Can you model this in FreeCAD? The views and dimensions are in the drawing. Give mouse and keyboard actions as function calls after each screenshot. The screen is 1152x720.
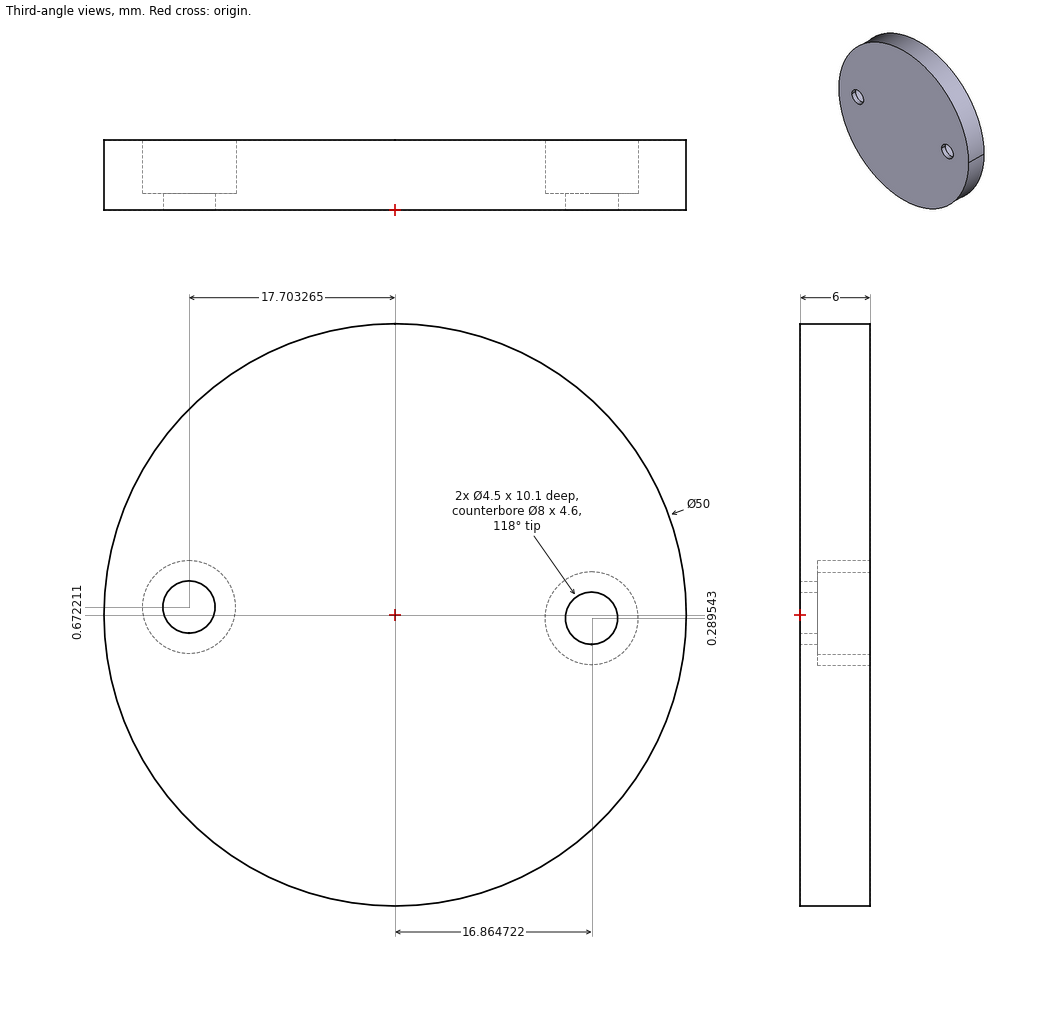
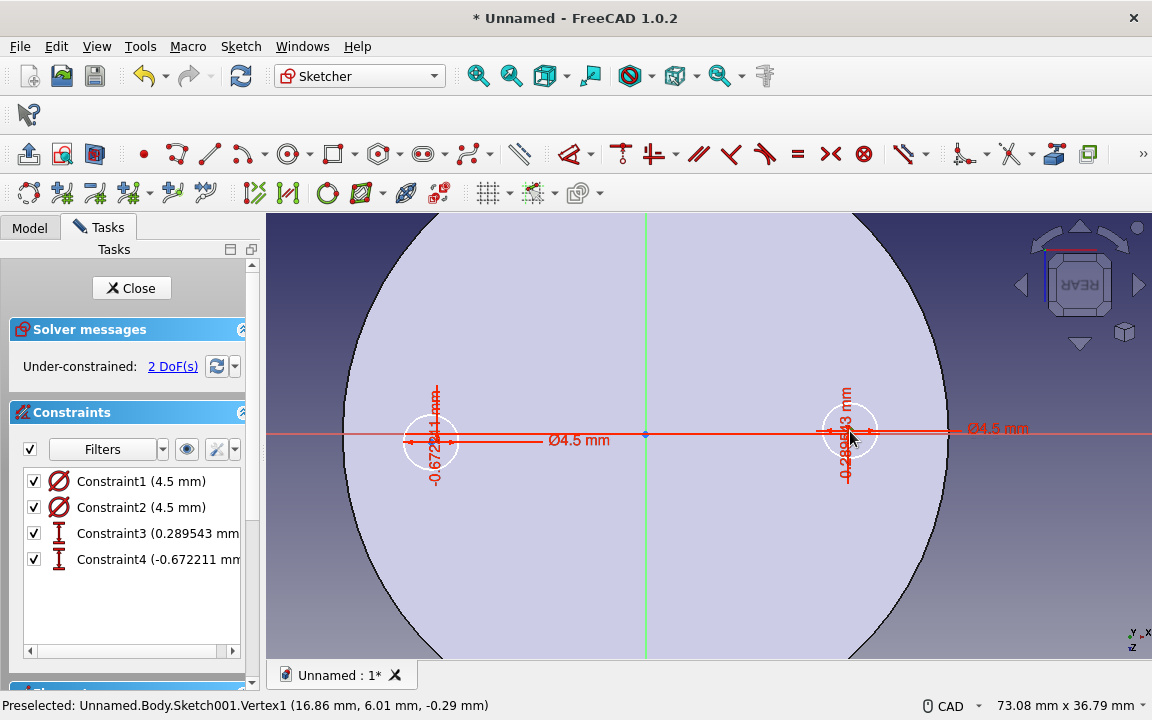
click(590, 154)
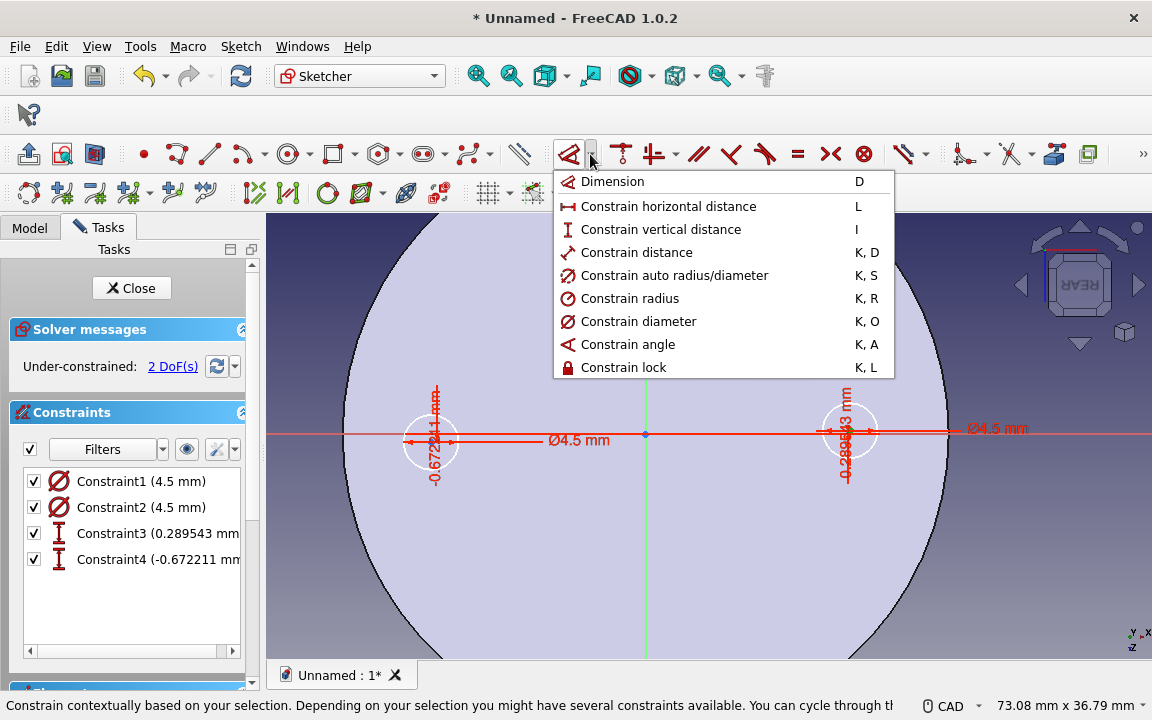
click(724, 206)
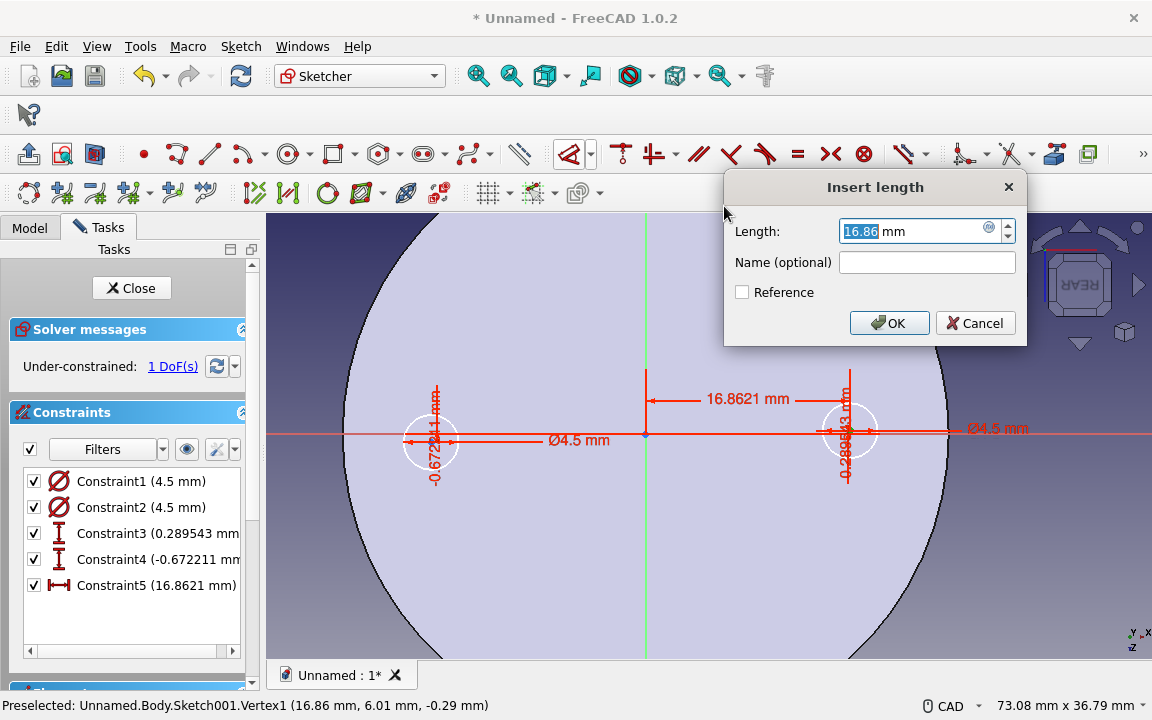
text(16.864722)
key(Return)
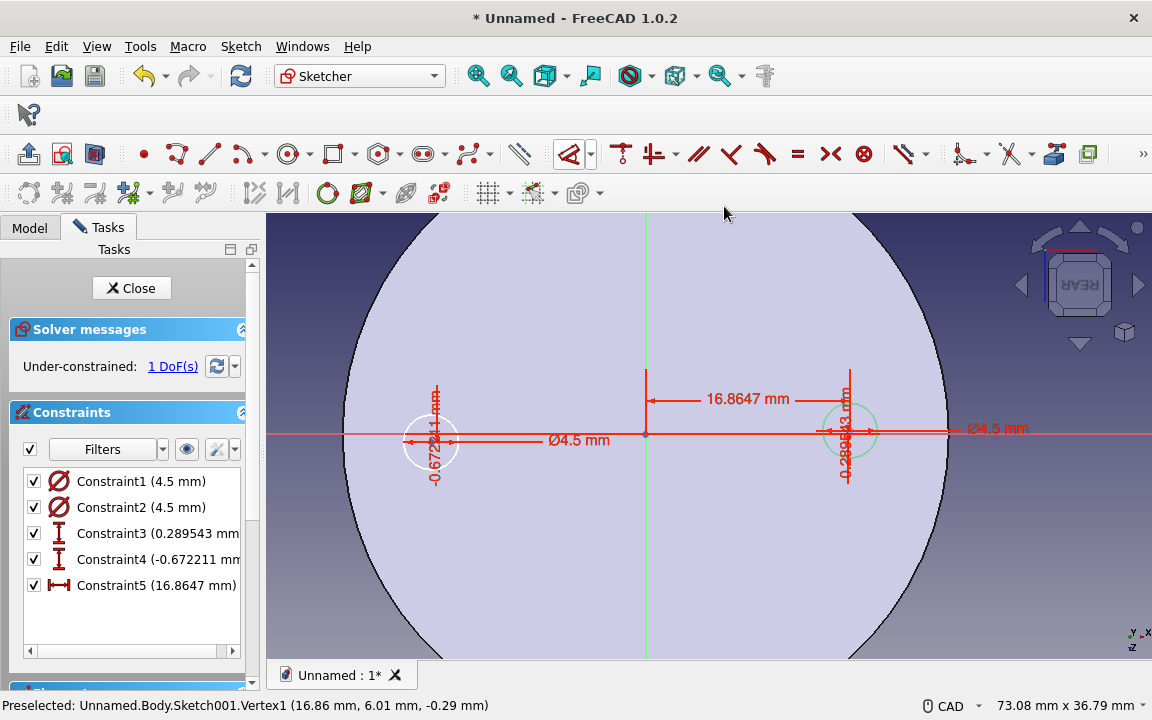
click(431, 442)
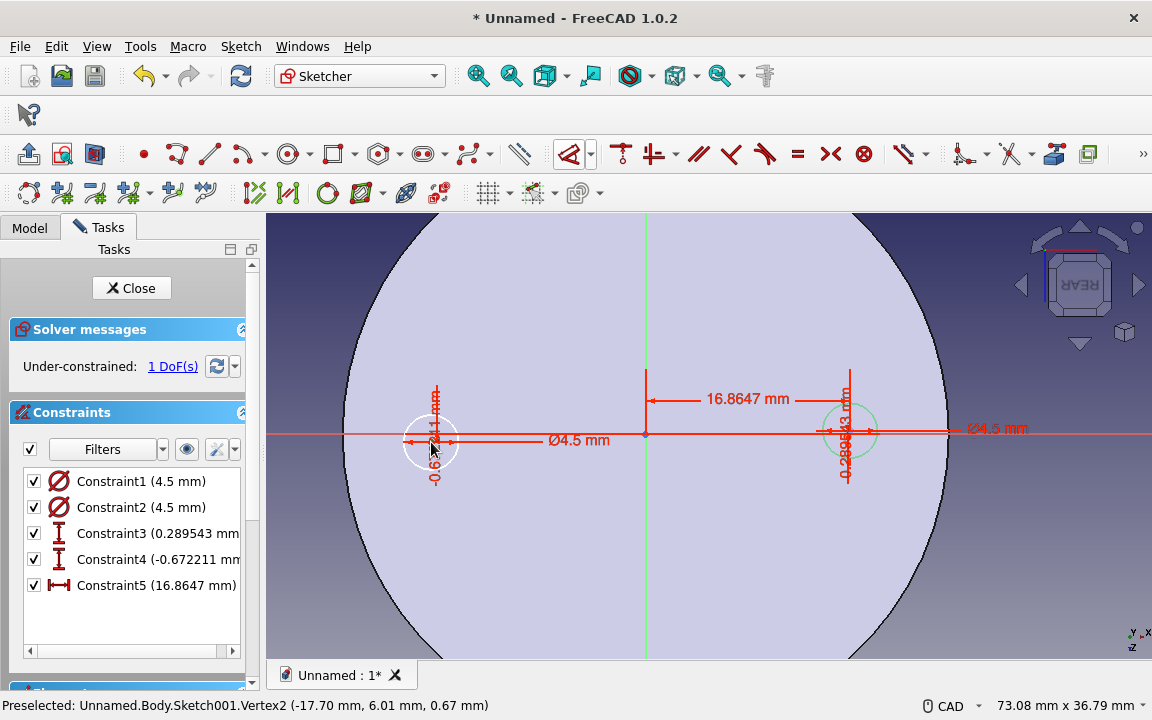
click(590, 154)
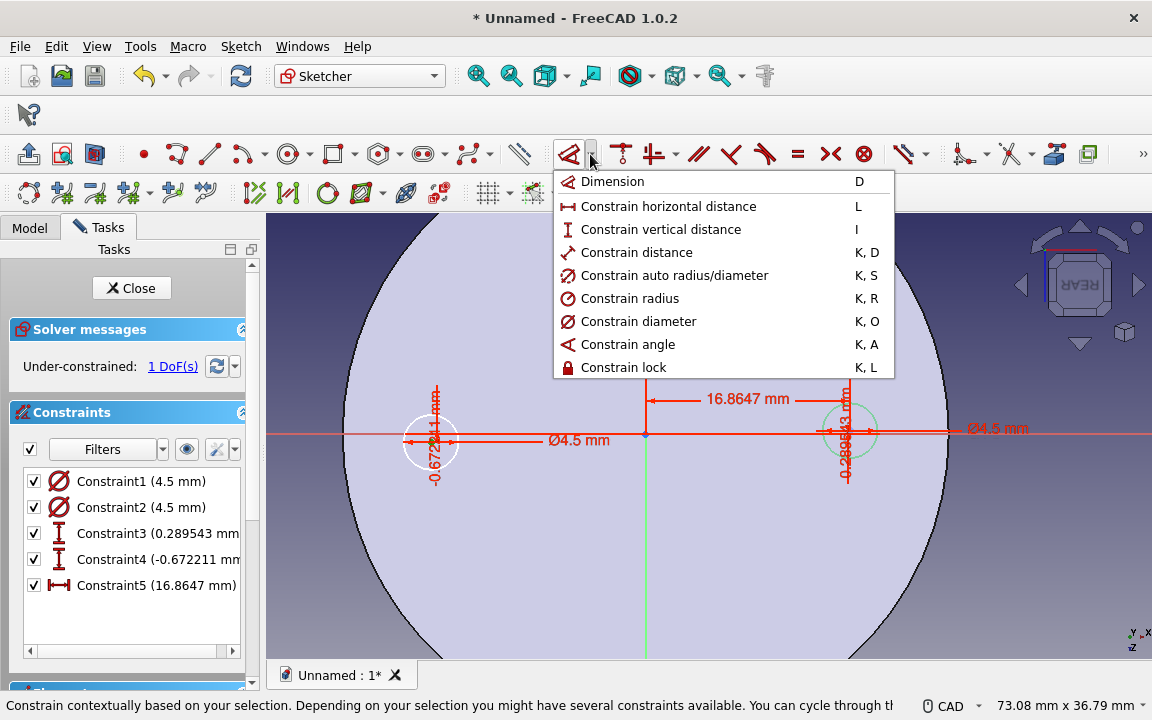
click(724, 206)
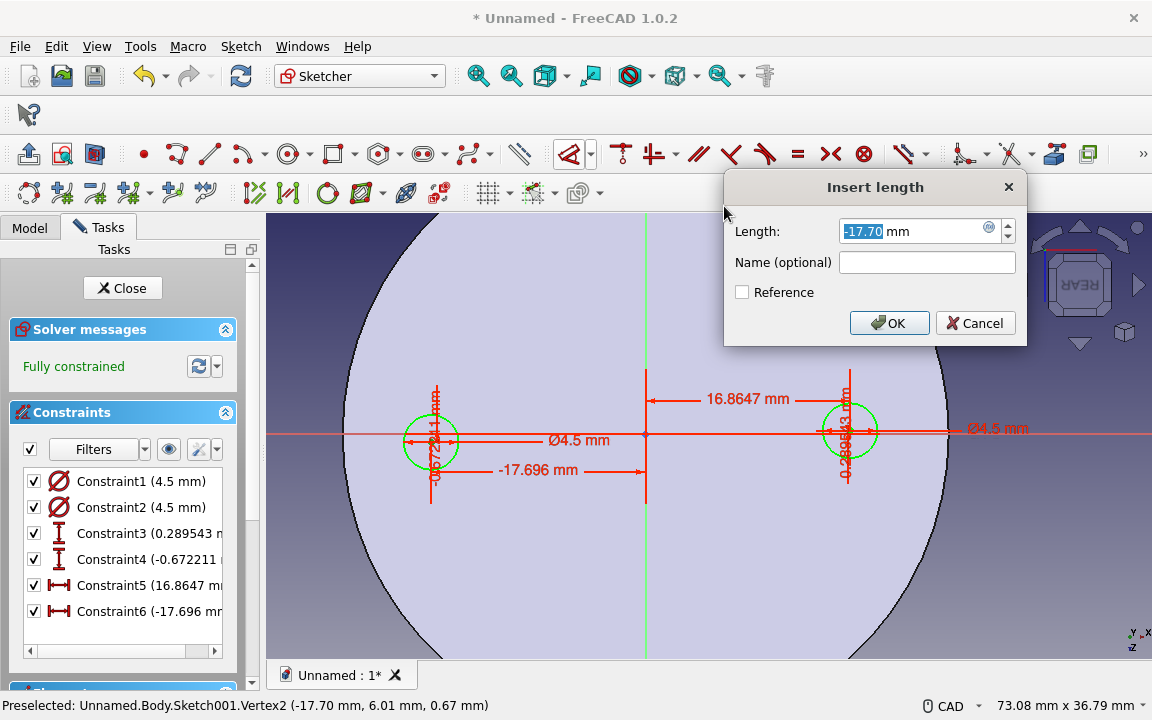
text(-17.703265)
key(Return)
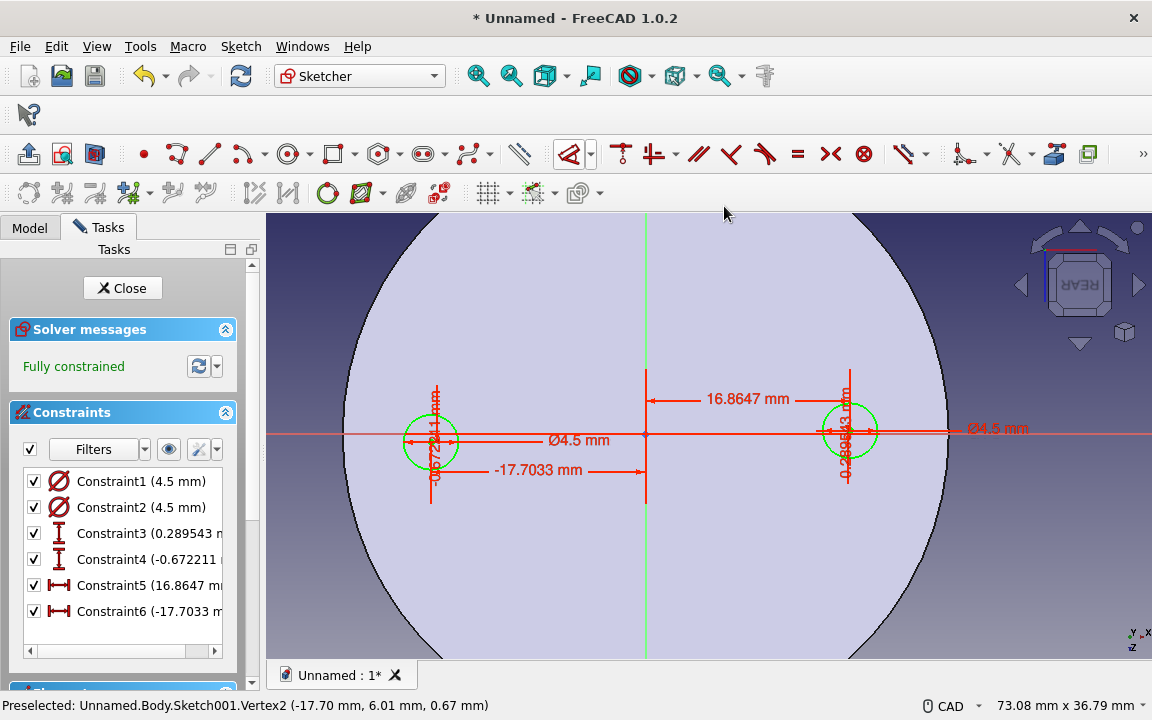
click(123, 288)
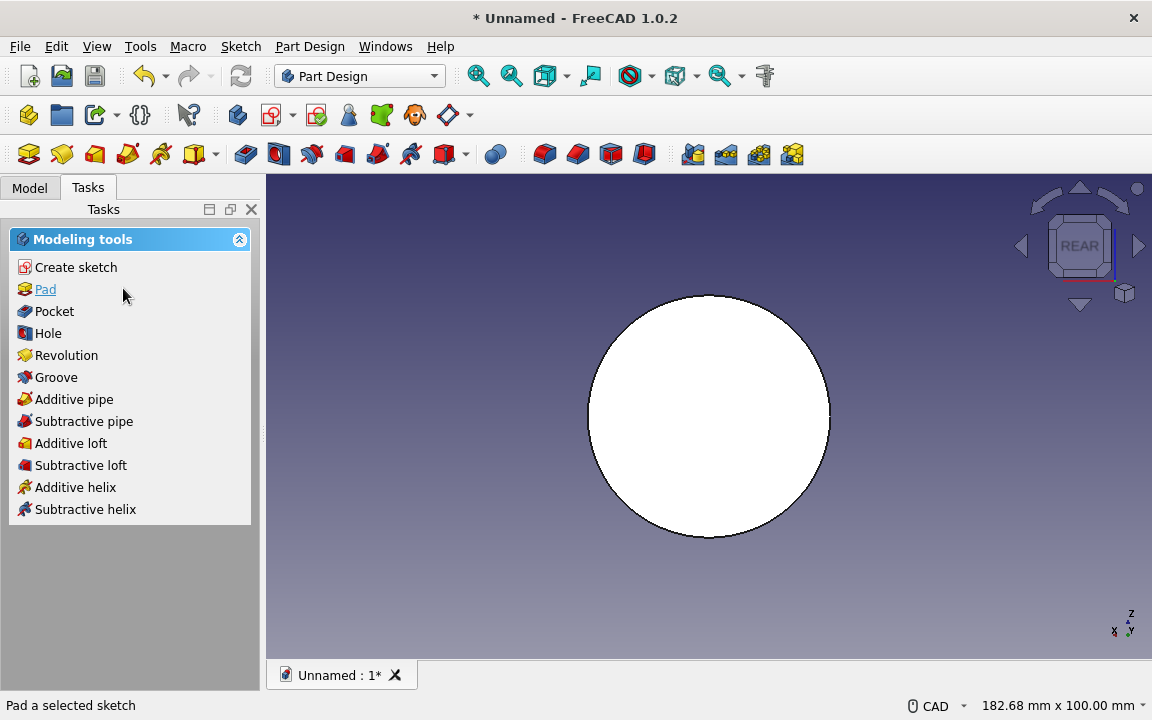
click(279, 154)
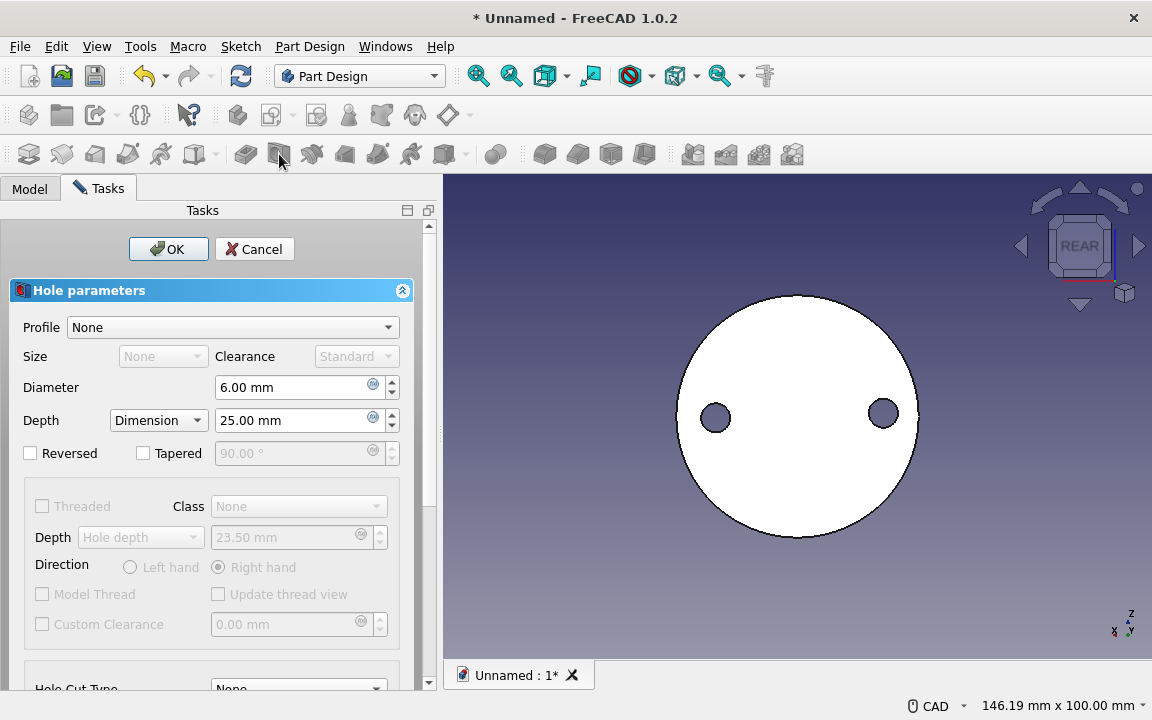
triple_click(300, 388)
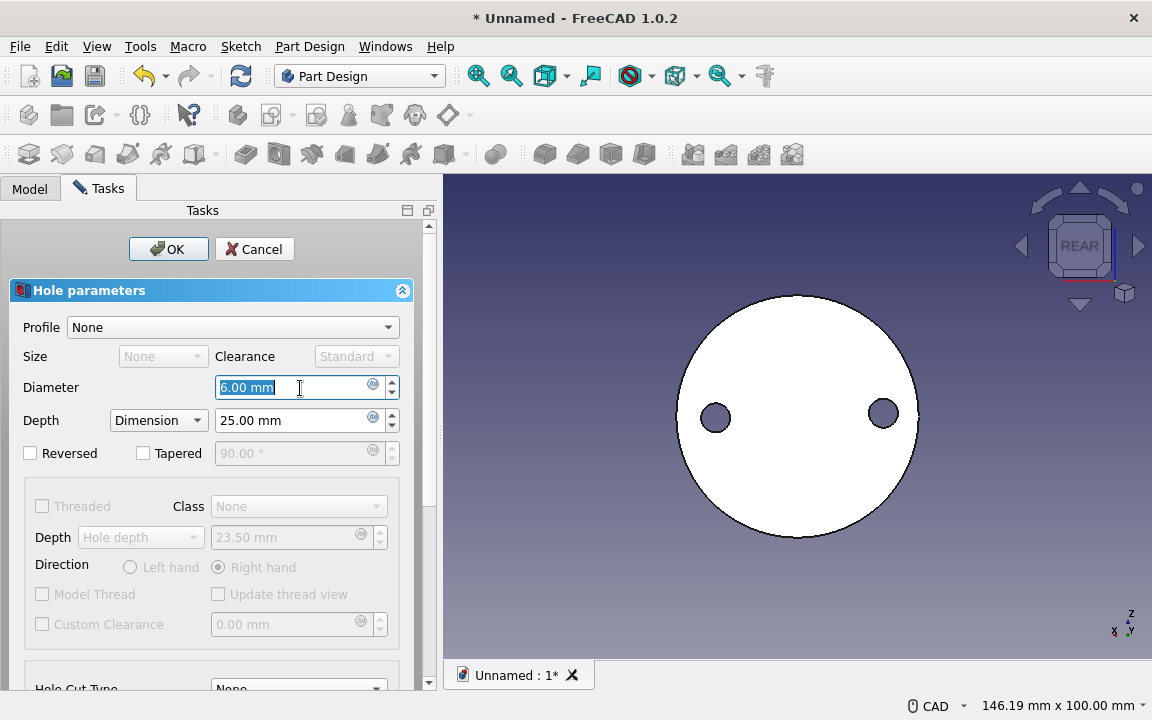
text(4.5)
key(Tab)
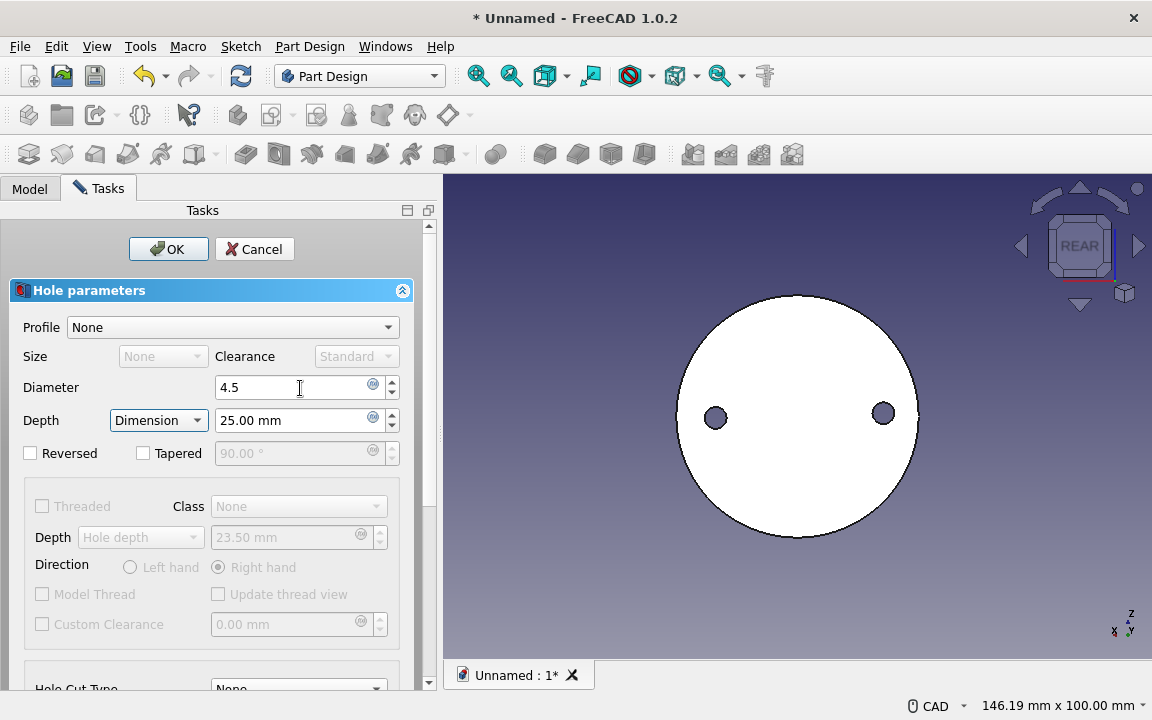
triple_click(300, 420)